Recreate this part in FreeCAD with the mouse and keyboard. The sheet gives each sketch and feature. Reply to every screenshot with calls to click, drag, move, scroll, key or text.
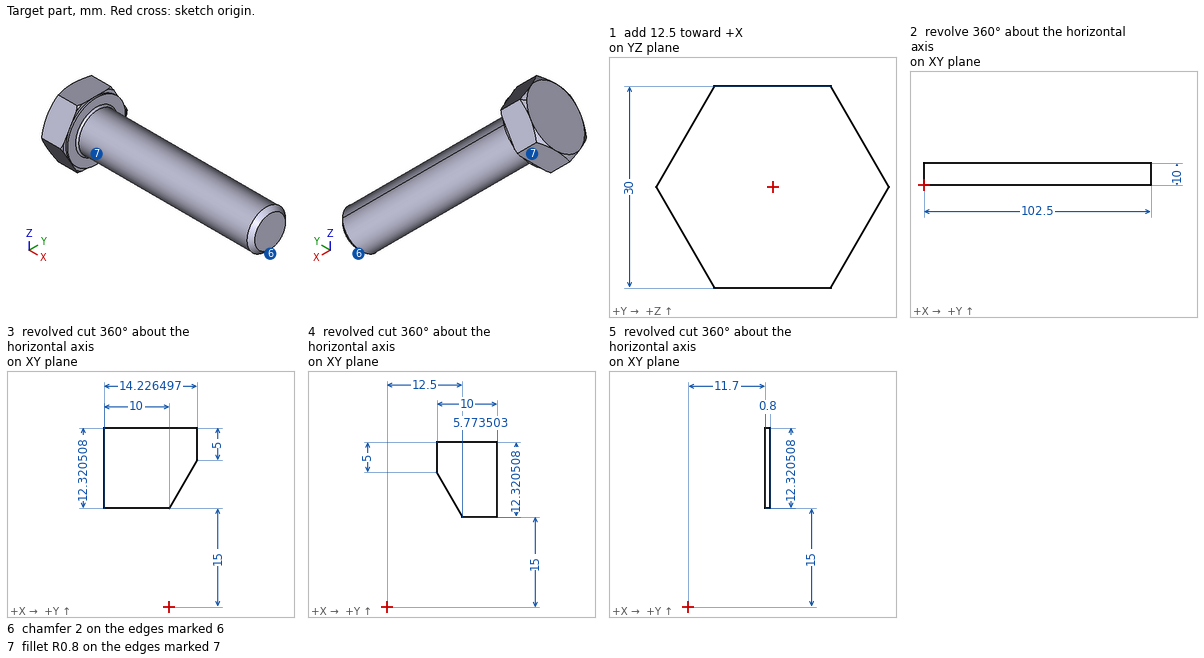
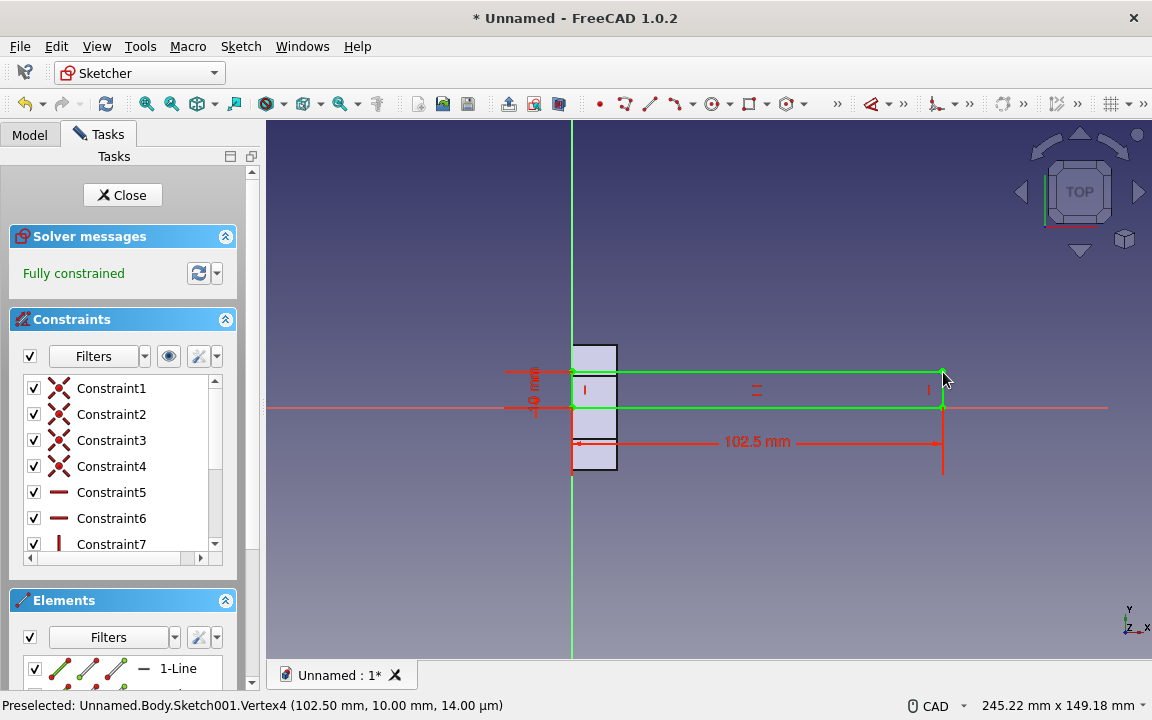
click(123, 195)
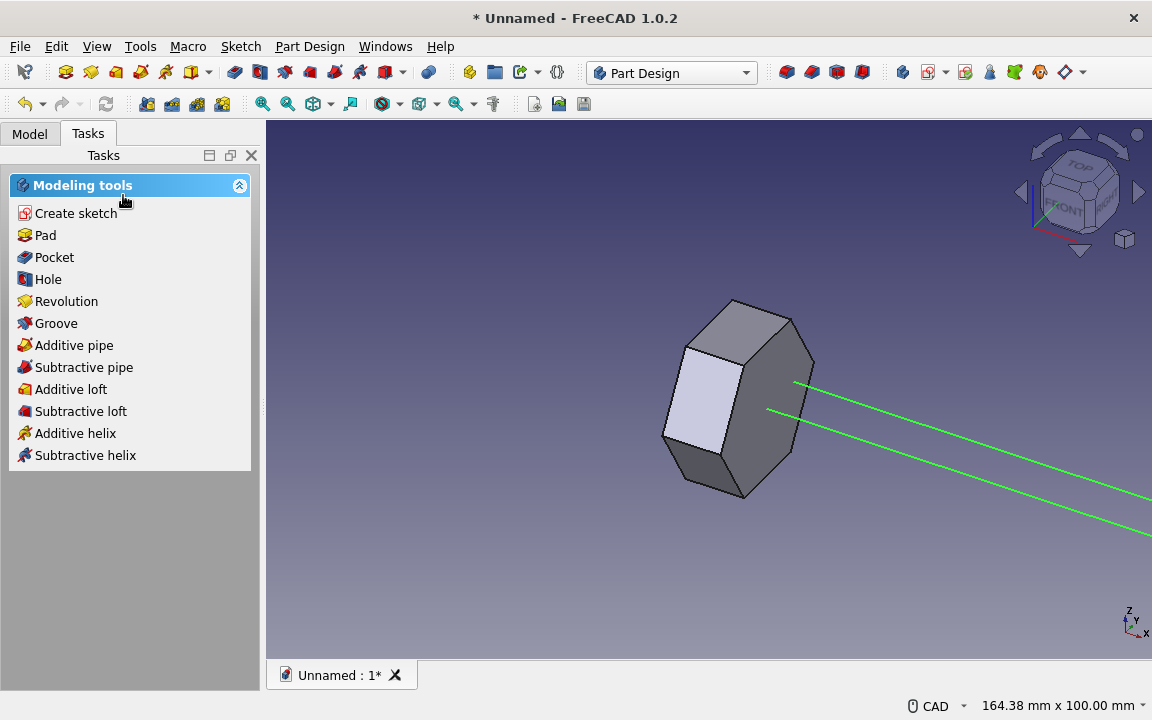
click(91, 72)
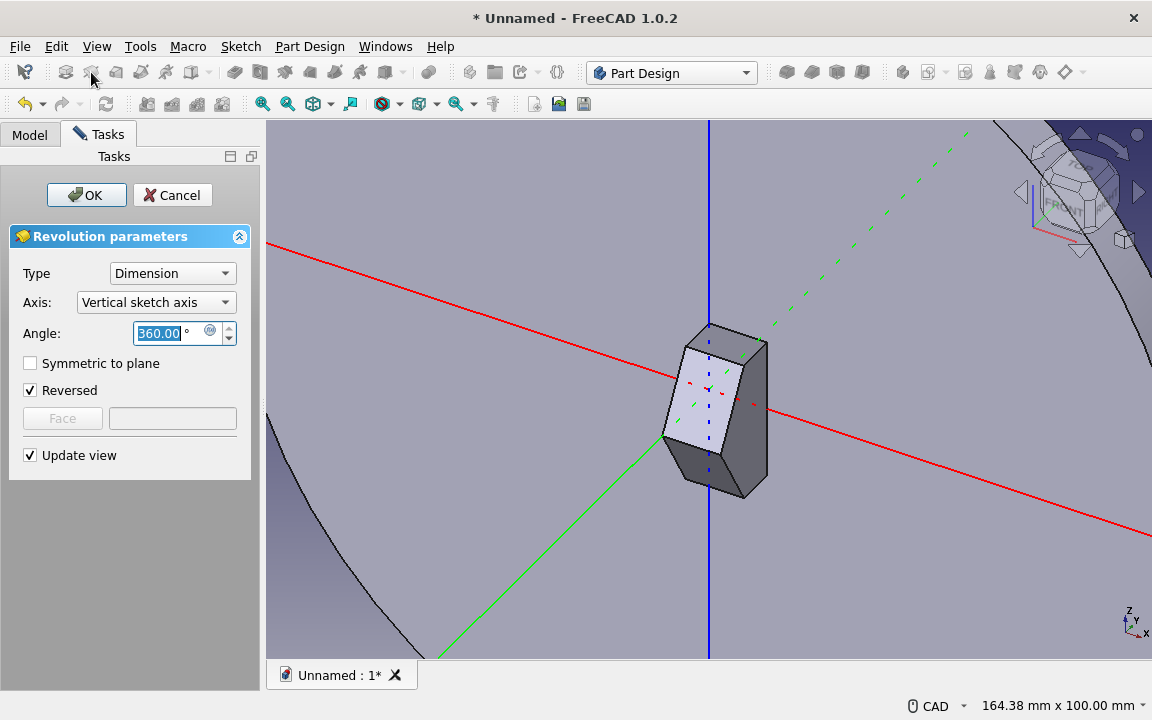
click(157, 302)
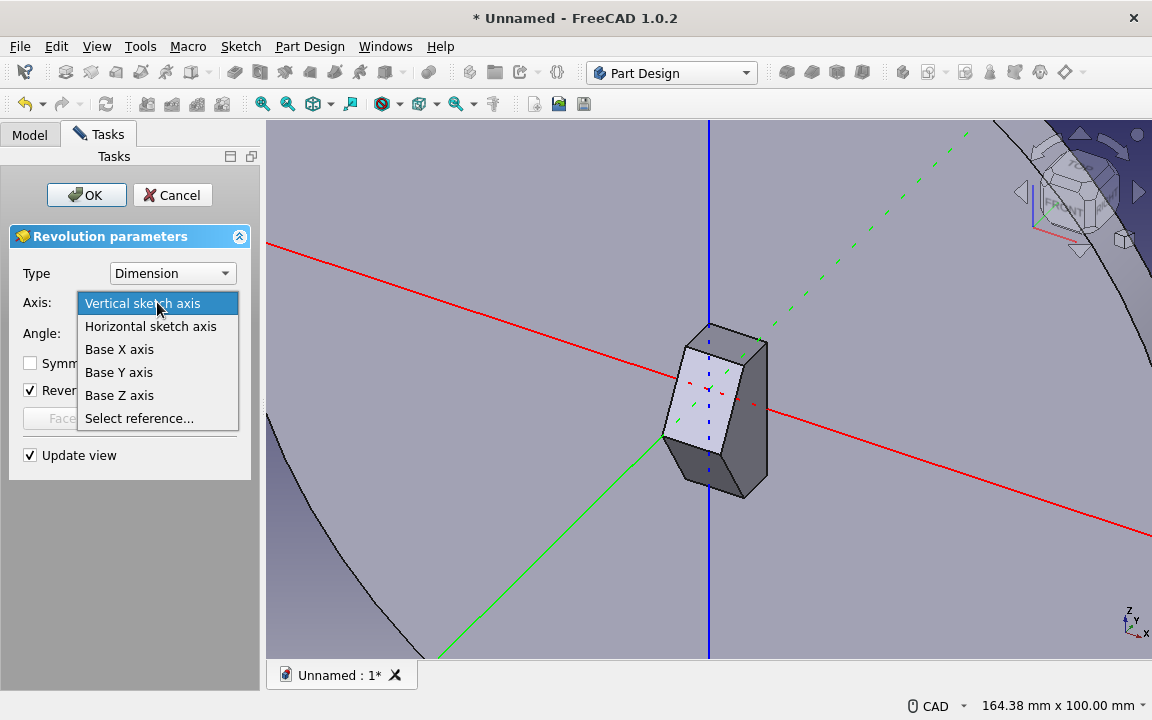
click(156, 326)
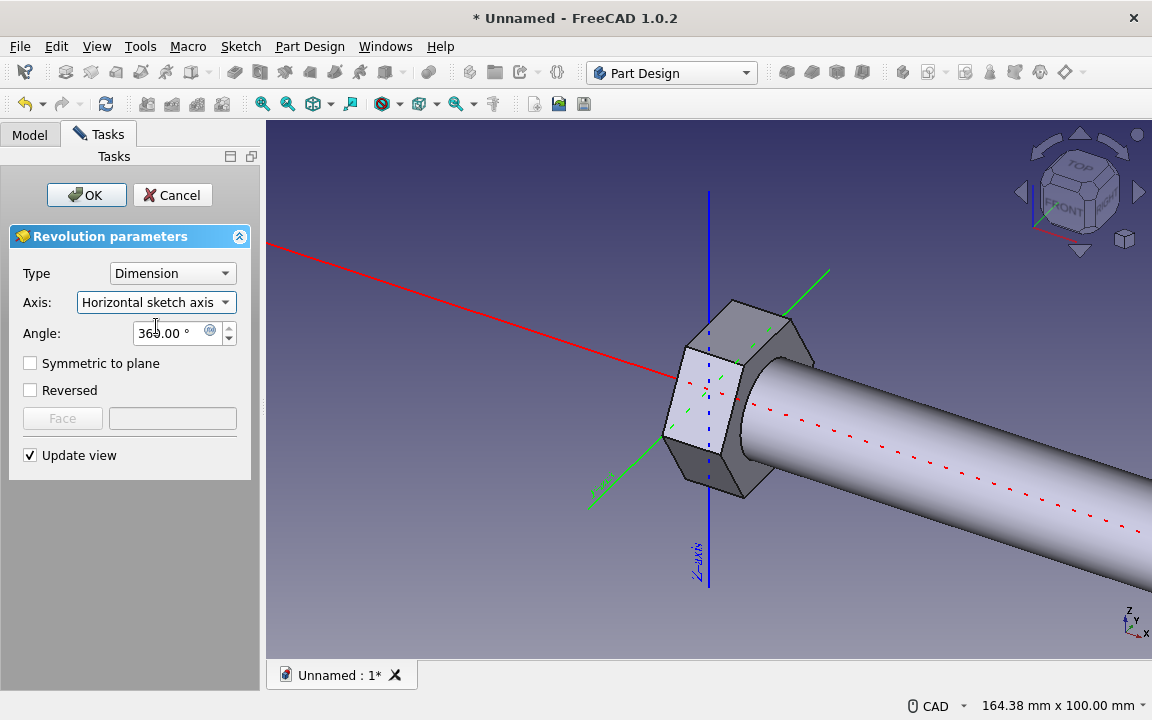
click(87, 195)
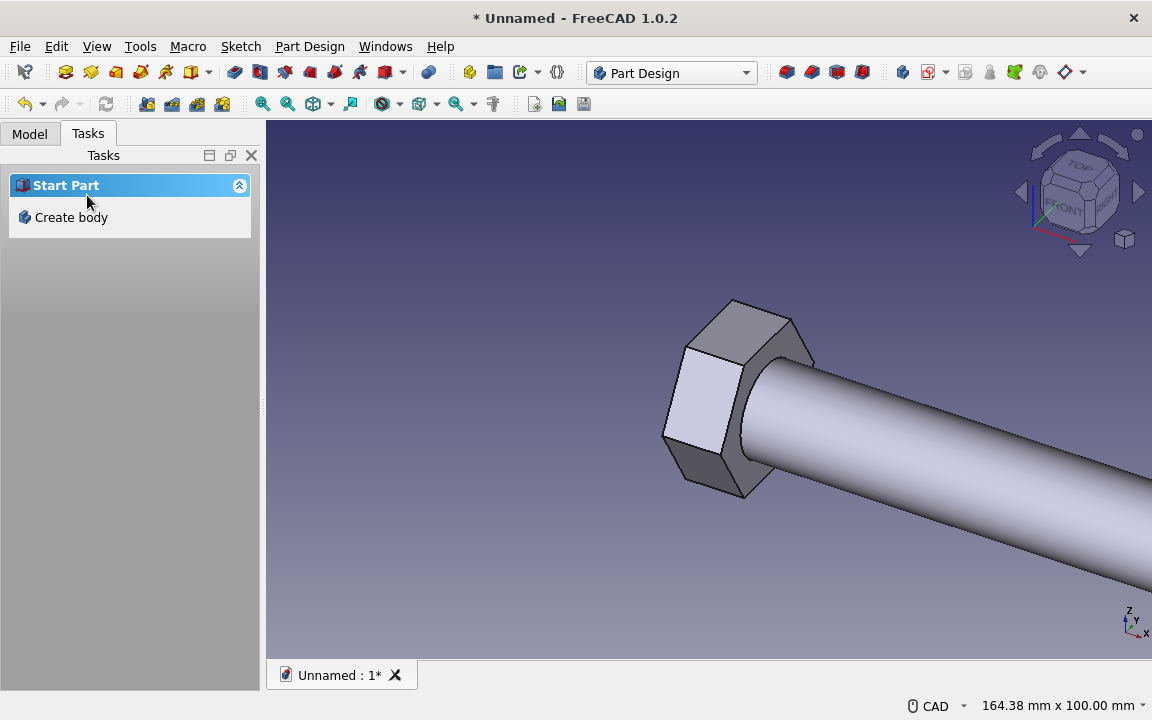
click(263, 104)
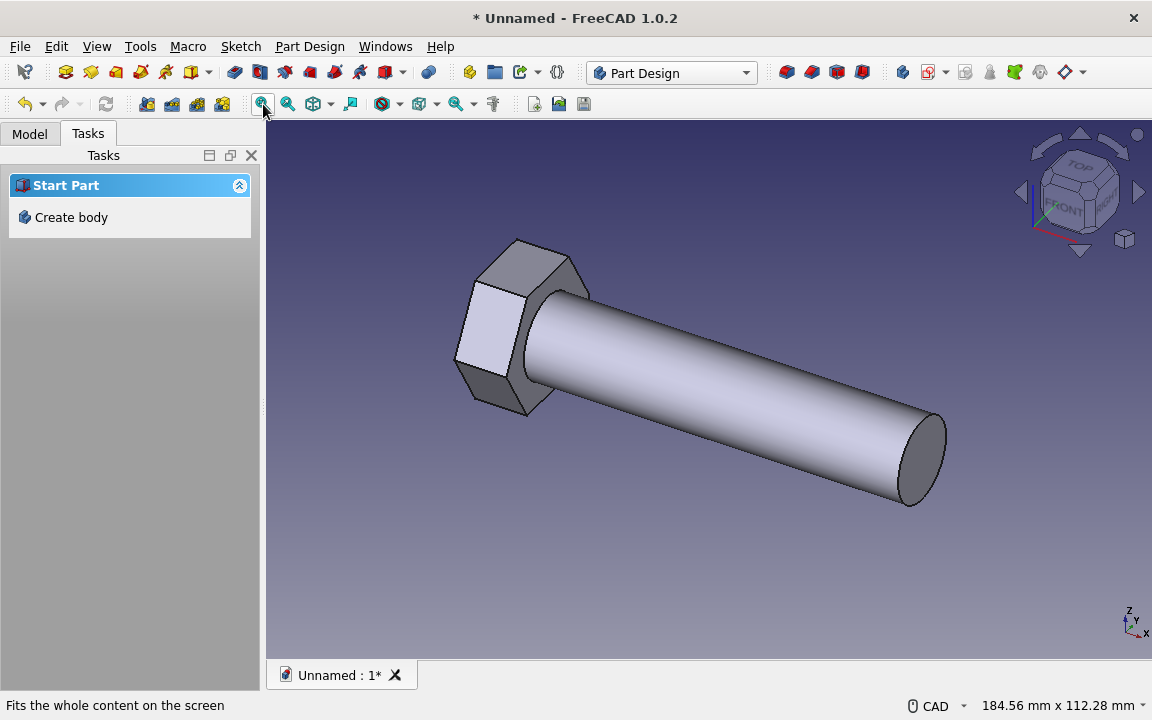
click(928, 72)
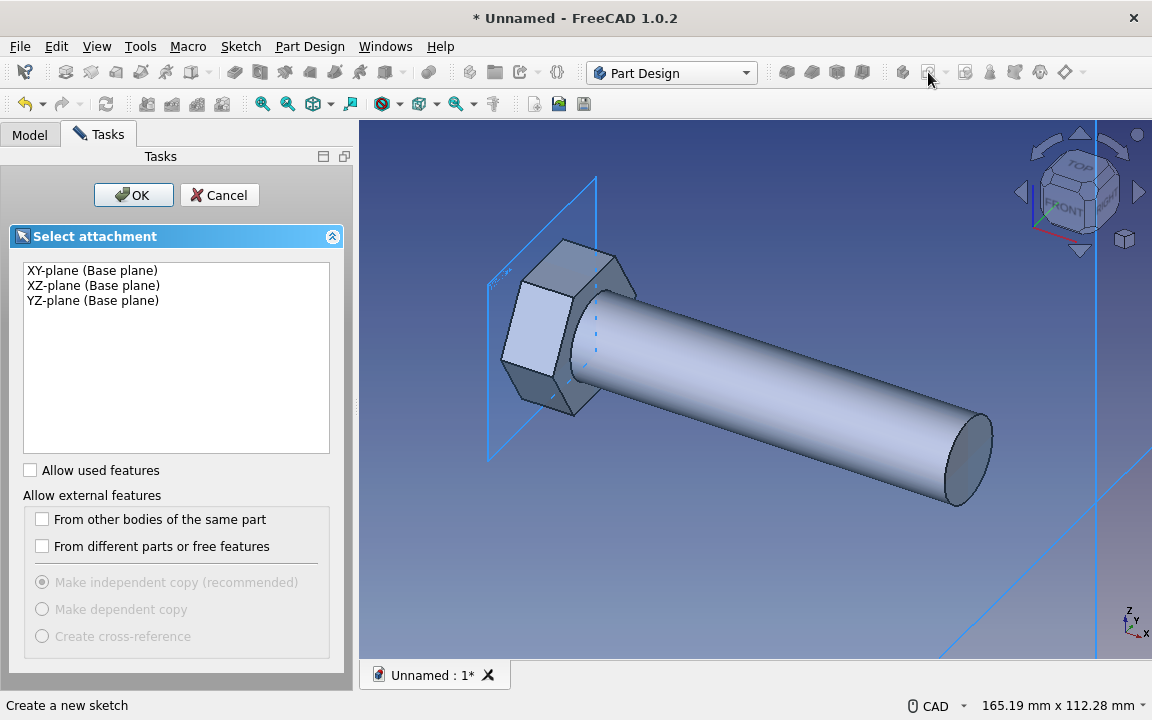
click(84, 270)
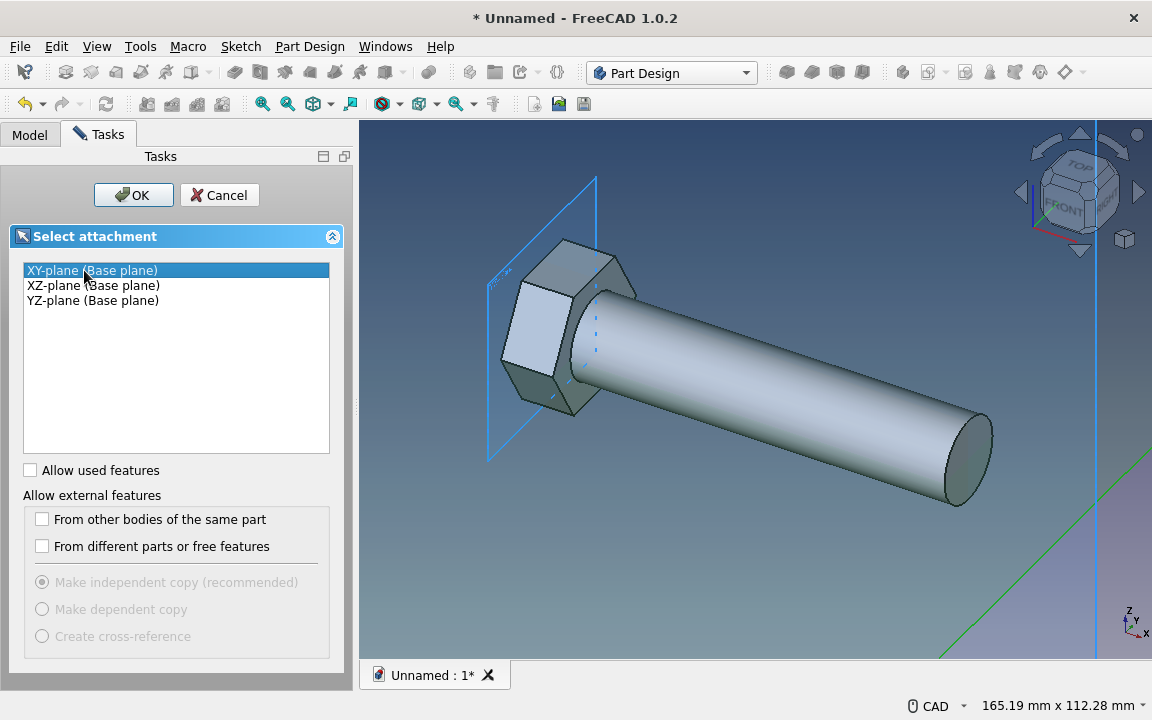
click(134, 195)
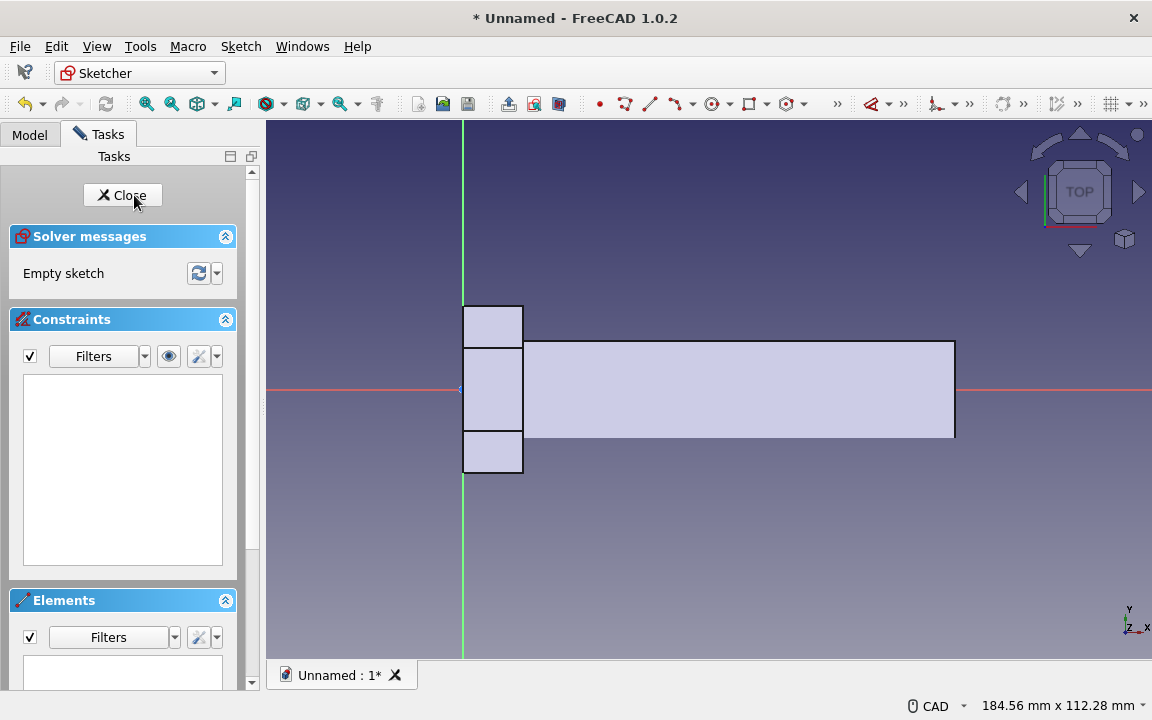
click(559, 104)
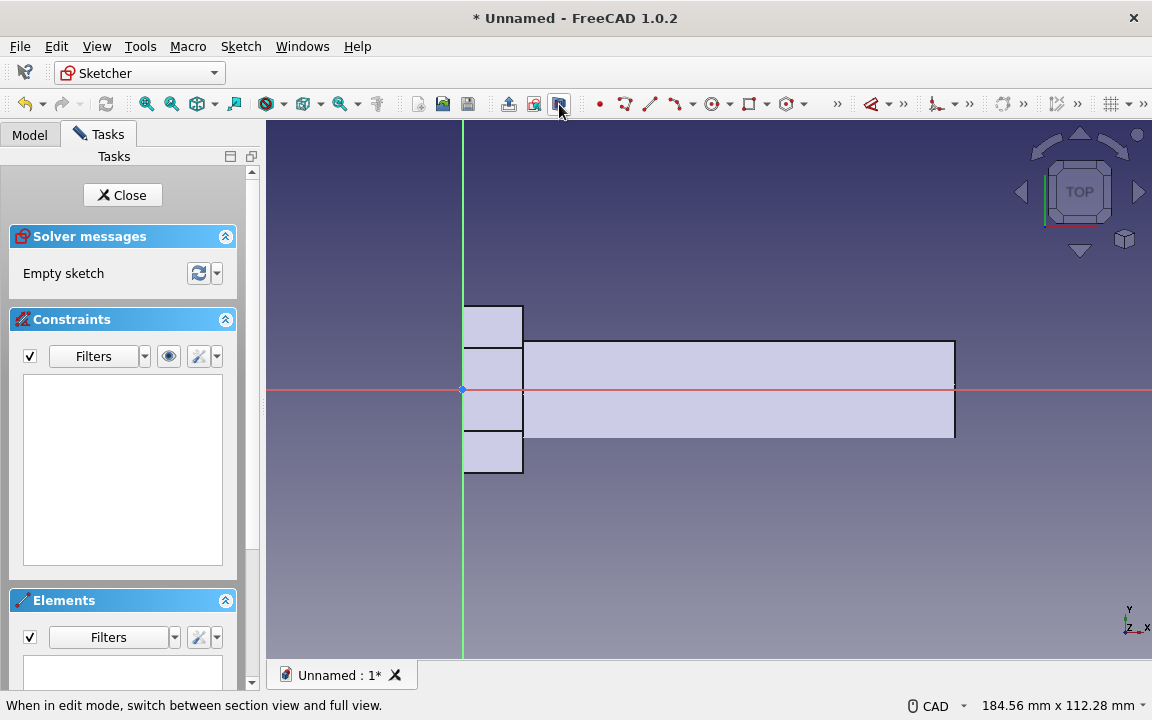
scroll(338, 286, up, 5)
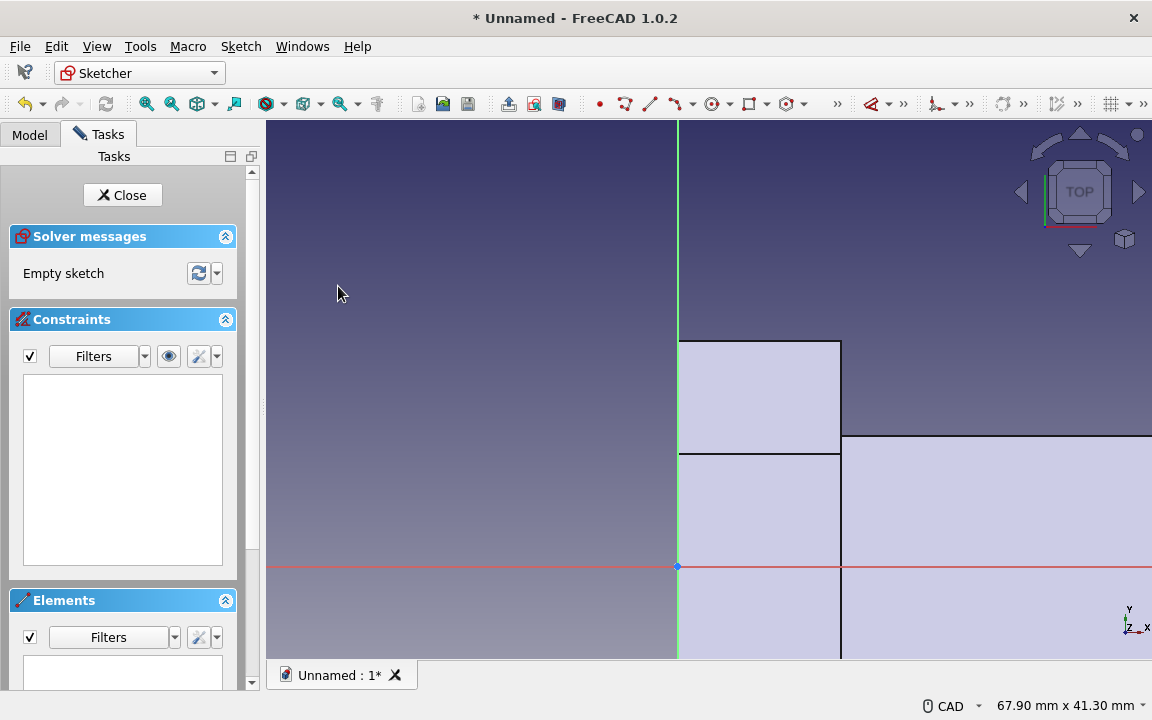
click(625, 104)